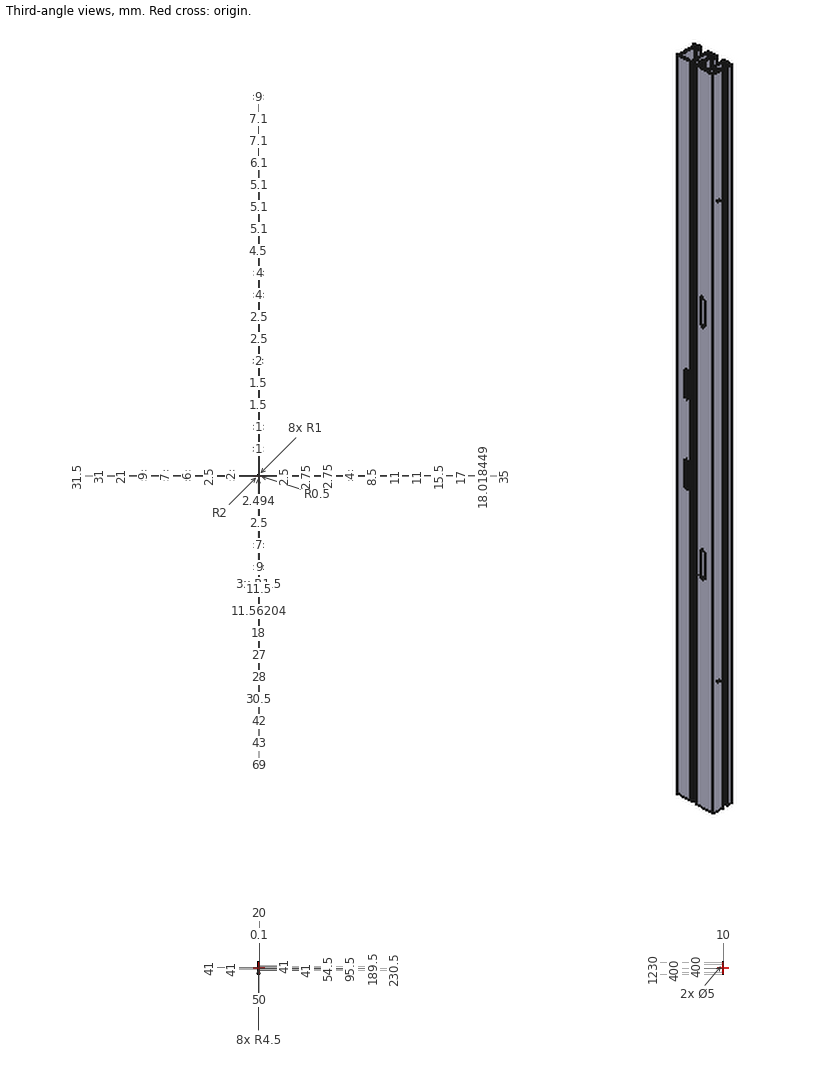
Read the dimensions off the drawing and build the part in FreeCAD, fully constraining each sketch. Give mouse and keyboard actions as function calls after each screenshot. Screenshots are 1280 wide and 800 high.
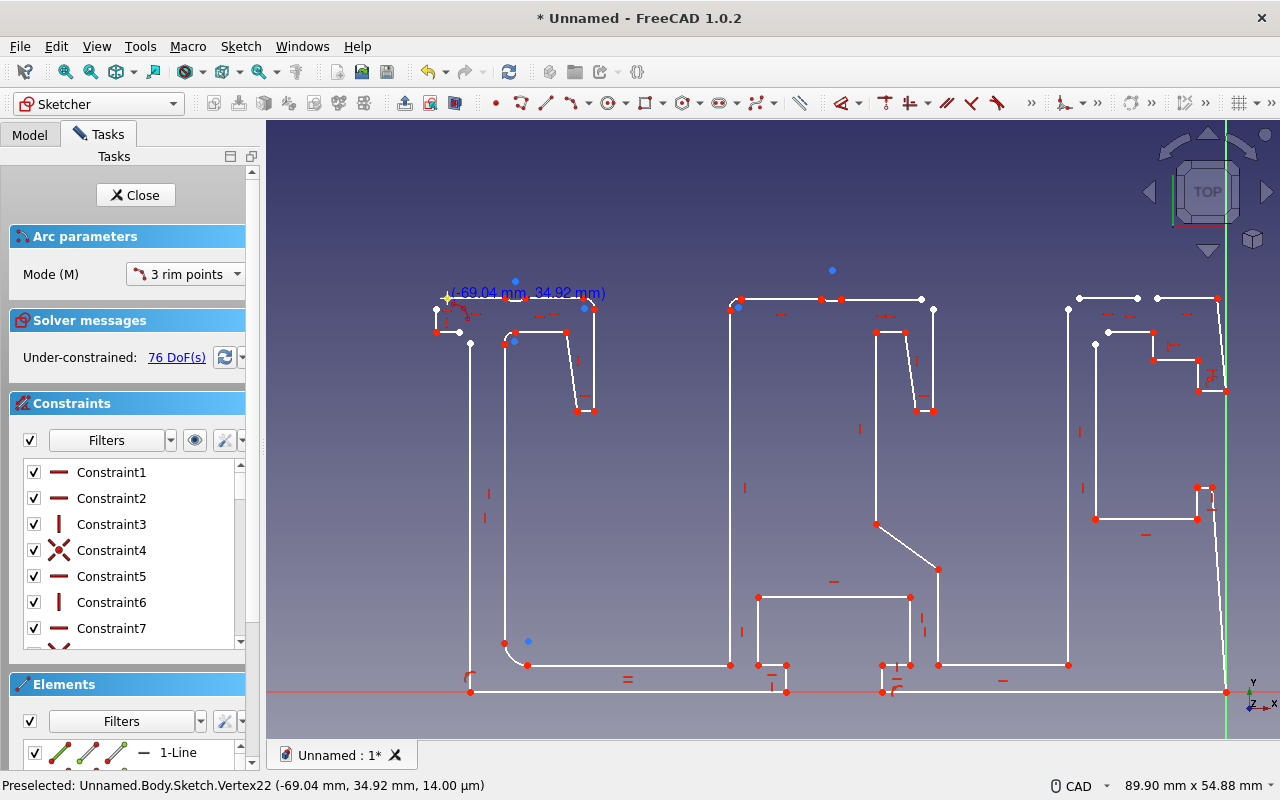
scroll(437, 309, up, 2)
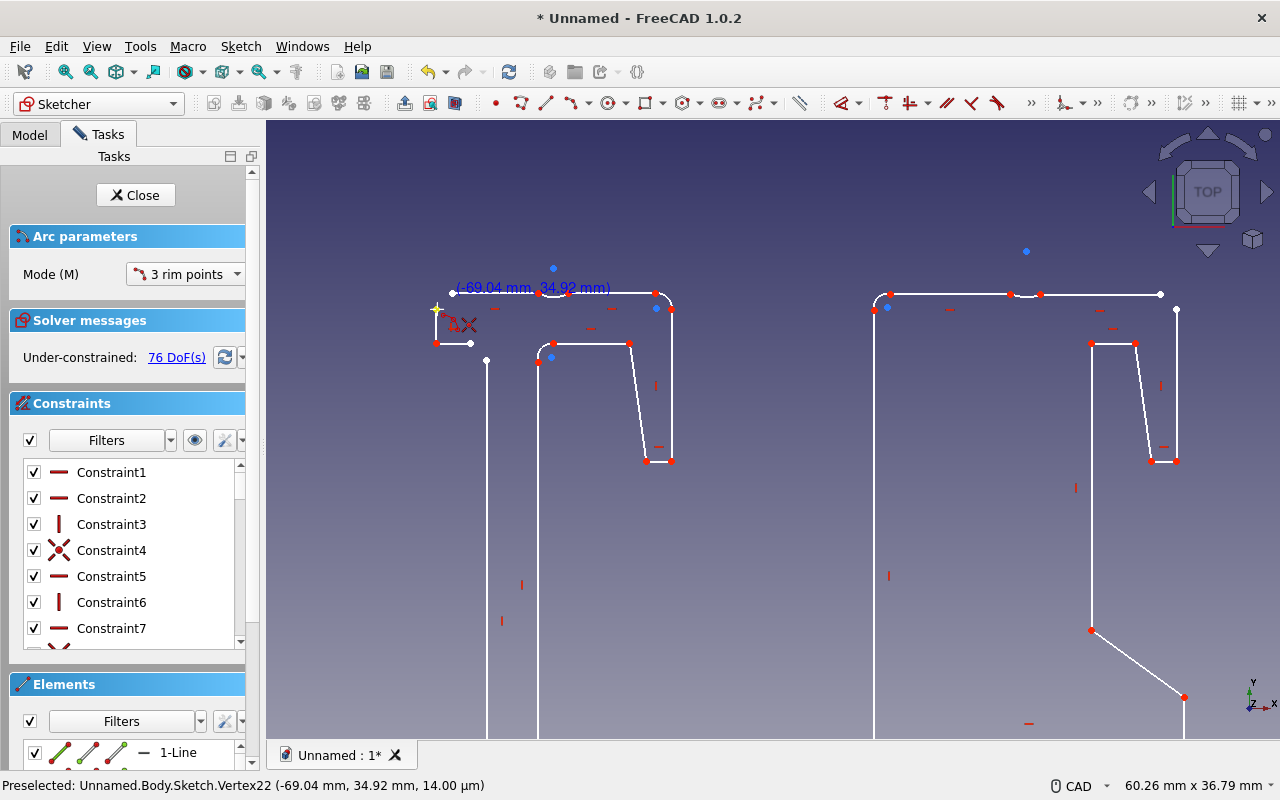
click(436, 309)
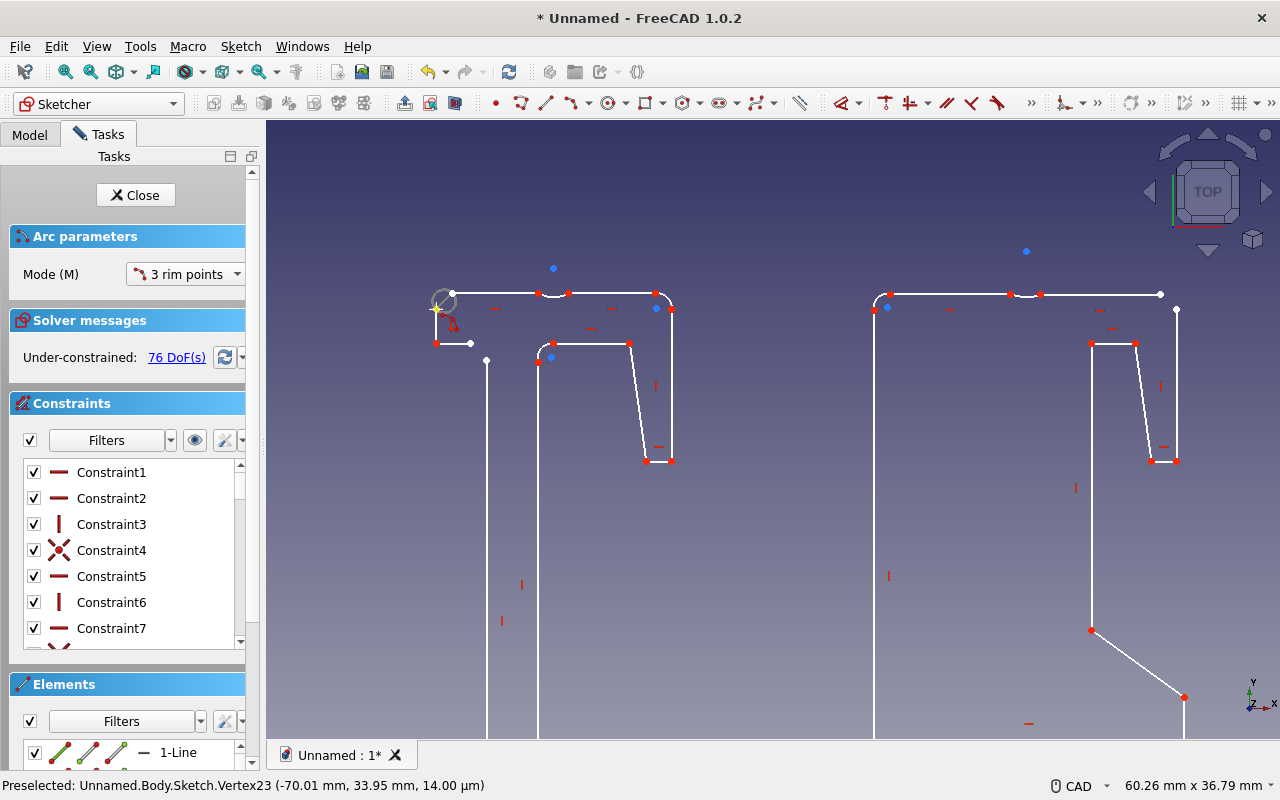
scroll(441, 297, up, 6)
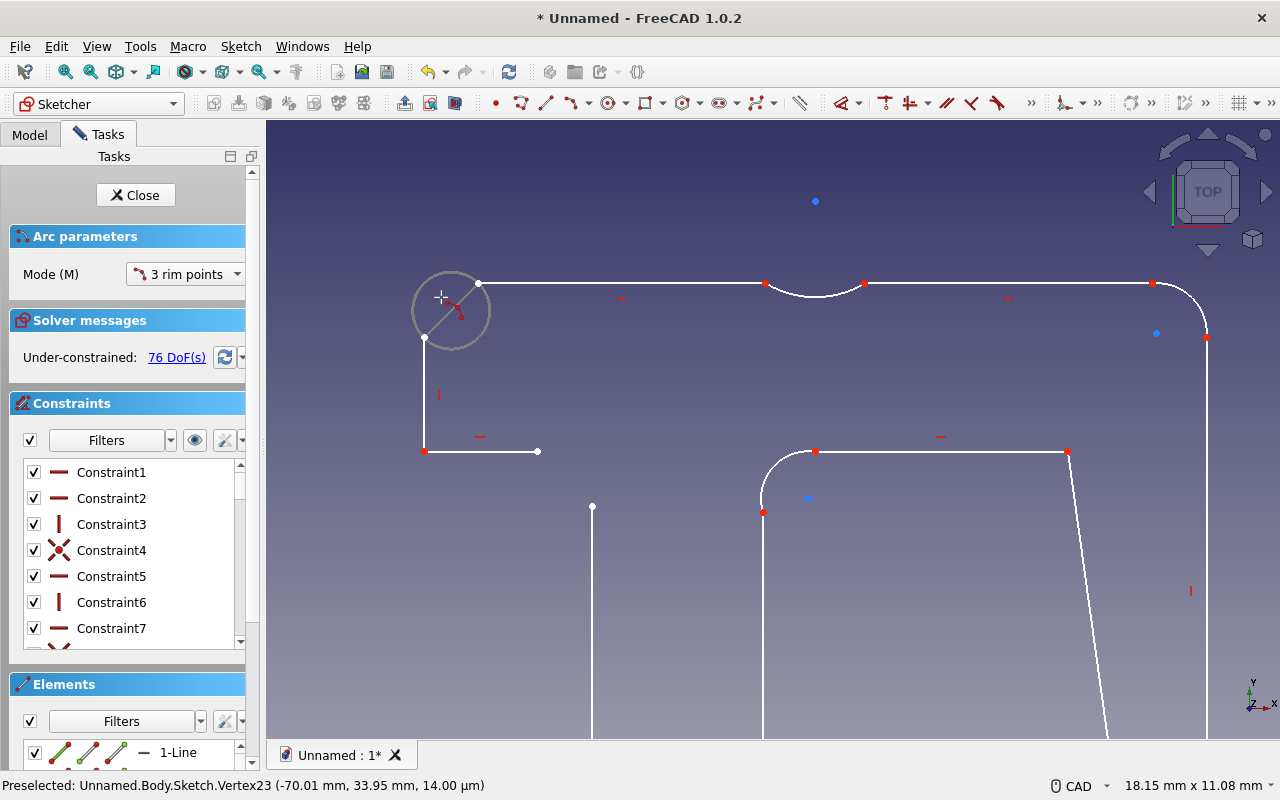
click(441, 295)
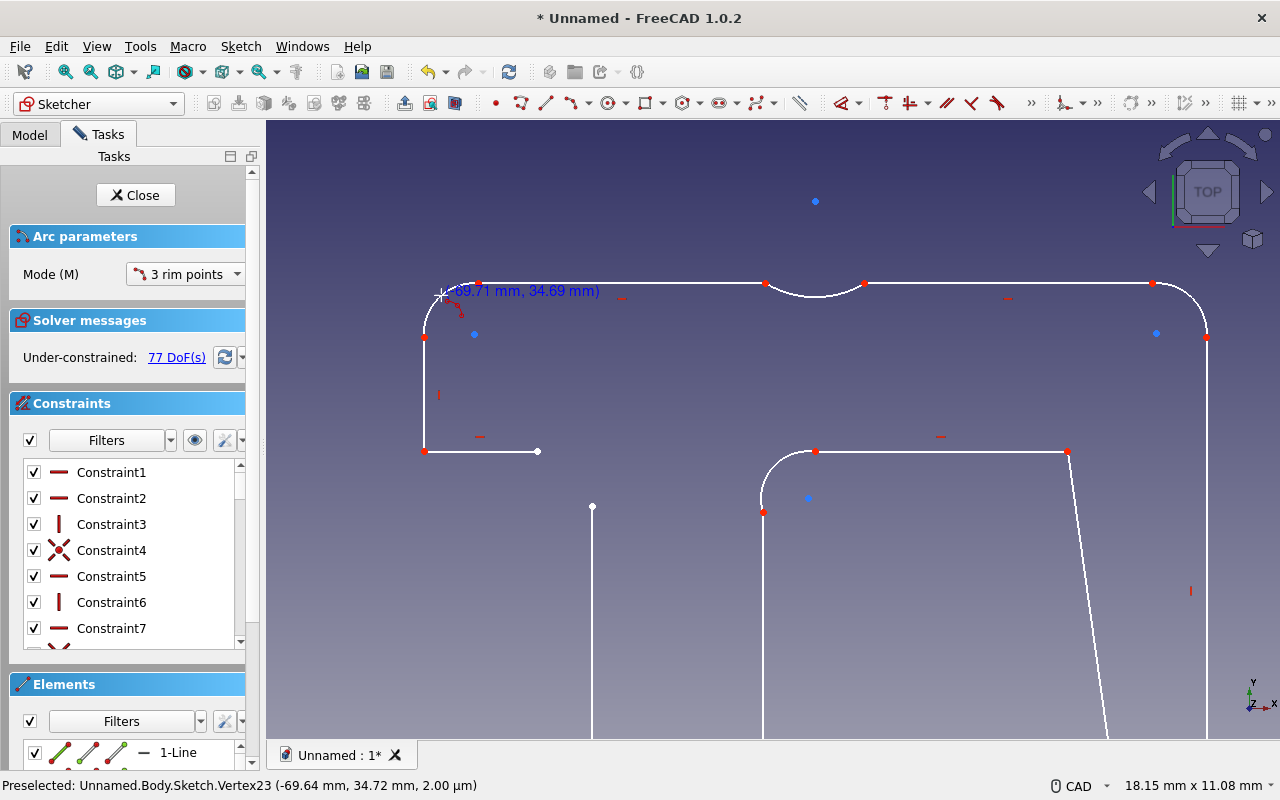
scroll(442, 300, down, 10)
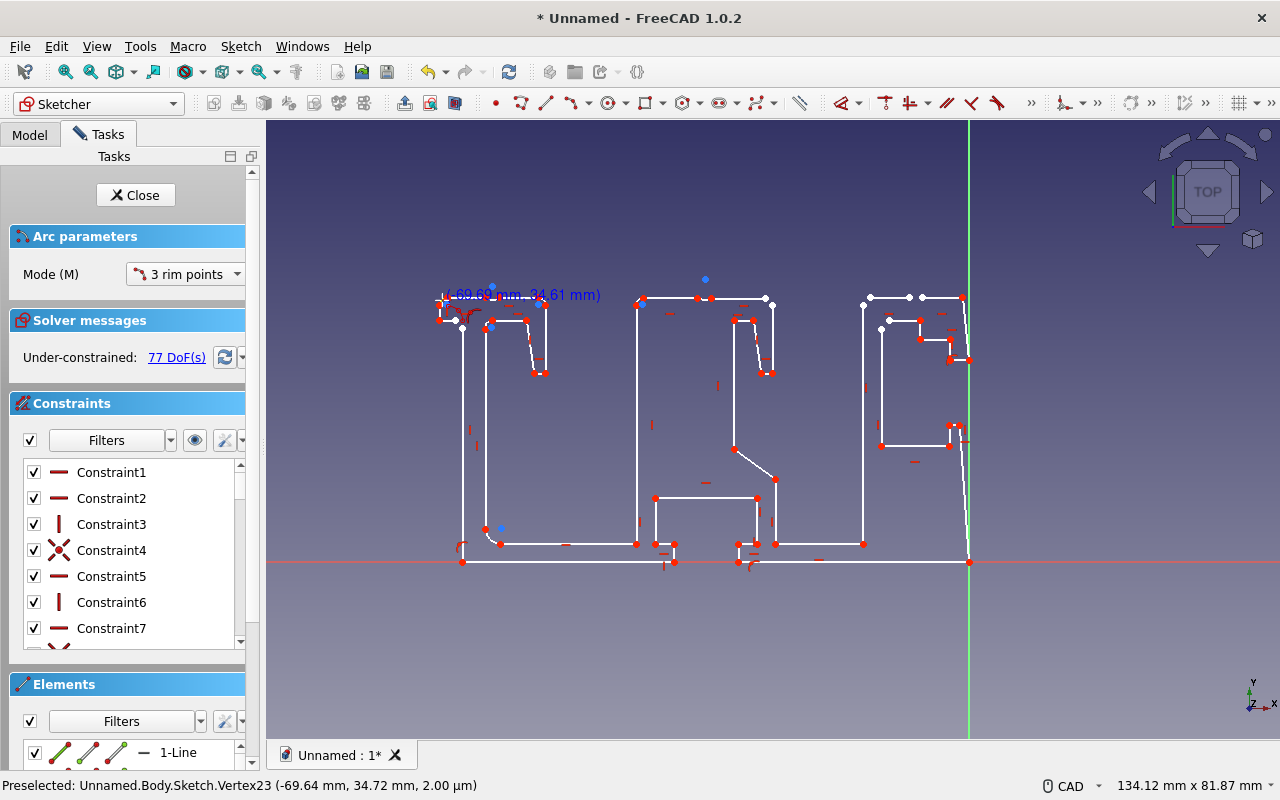
scroll(455, 320, up, 4)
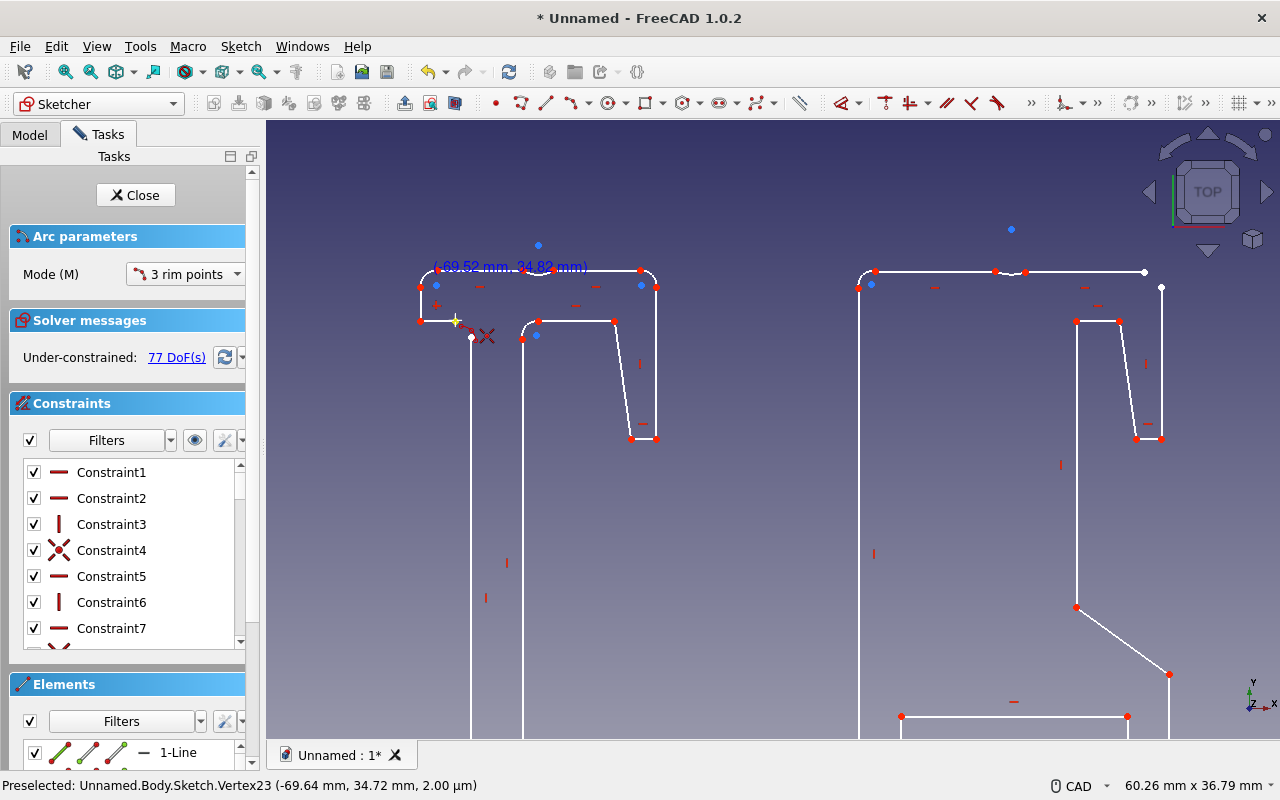
click(455, 321)
click(471, 338)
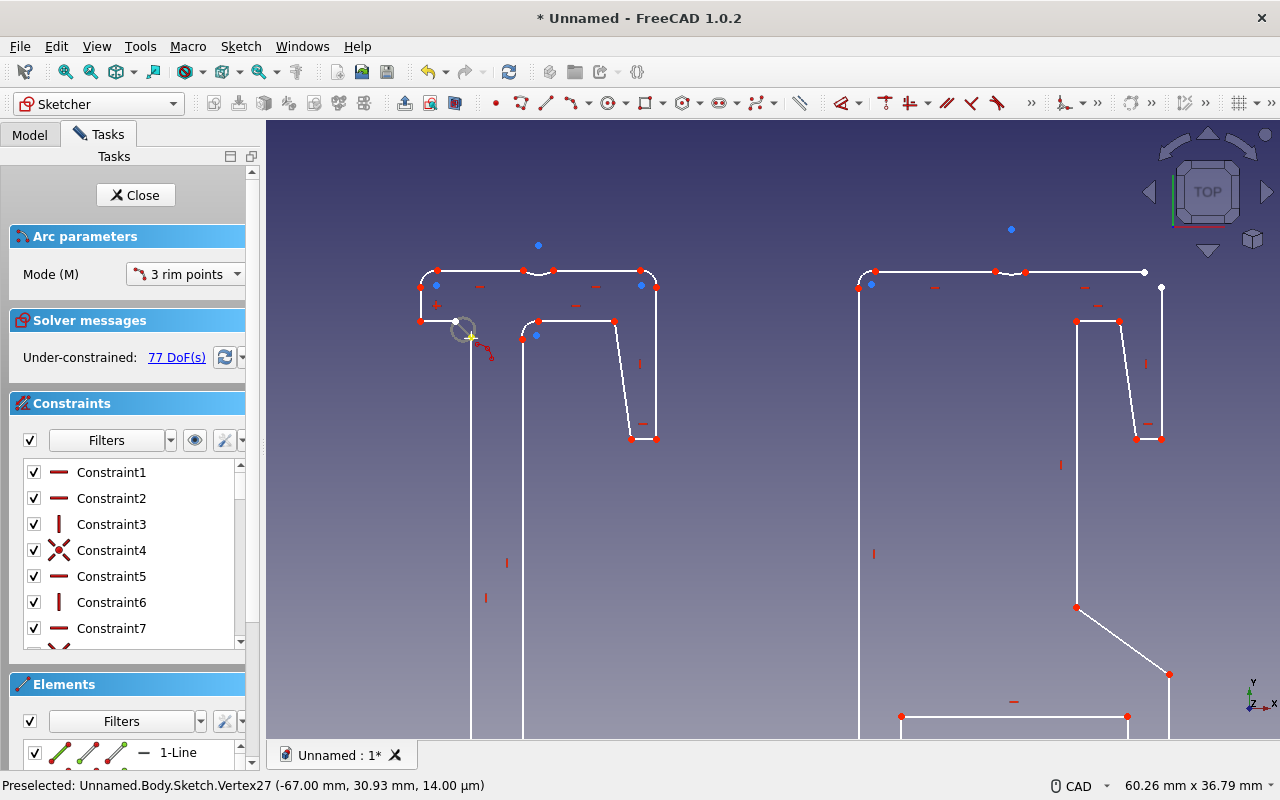
scroll(467, 325, up, 6)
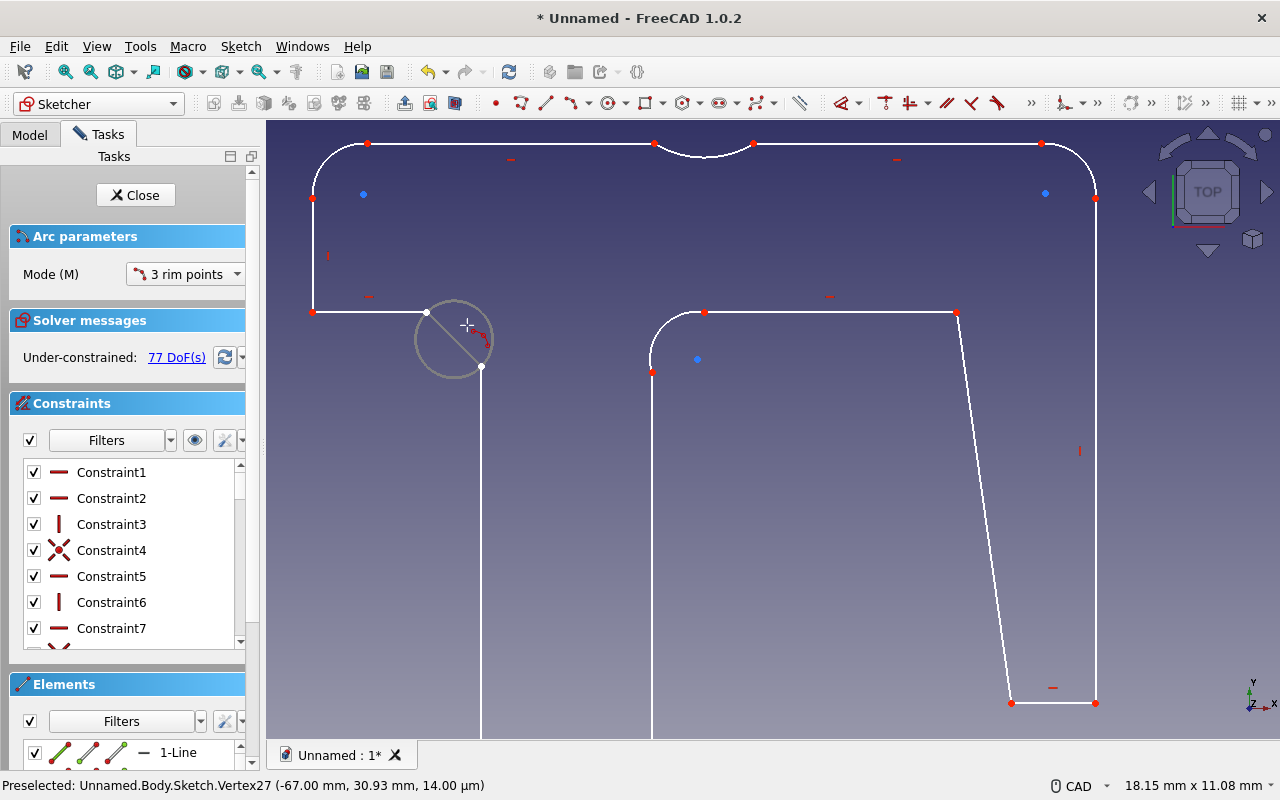
click(465, 323)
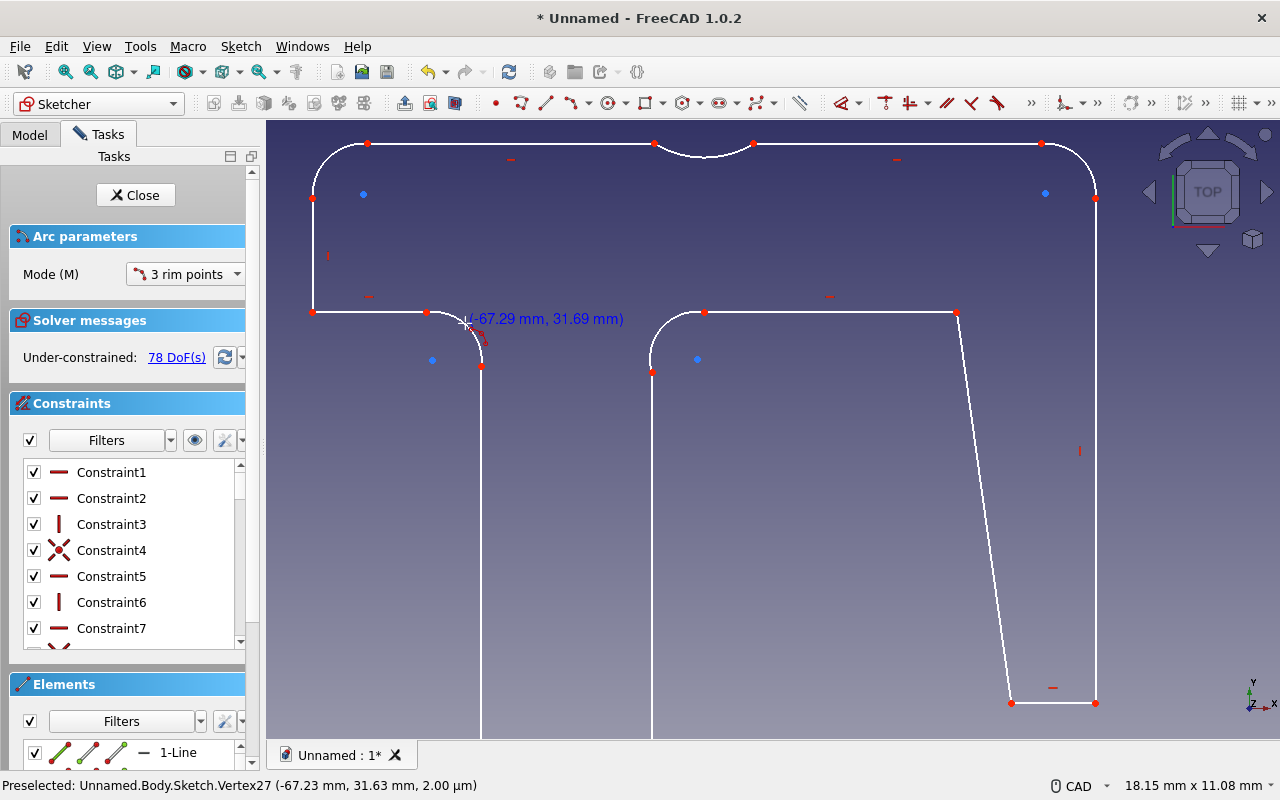
scroll(460, 322, down, 10)